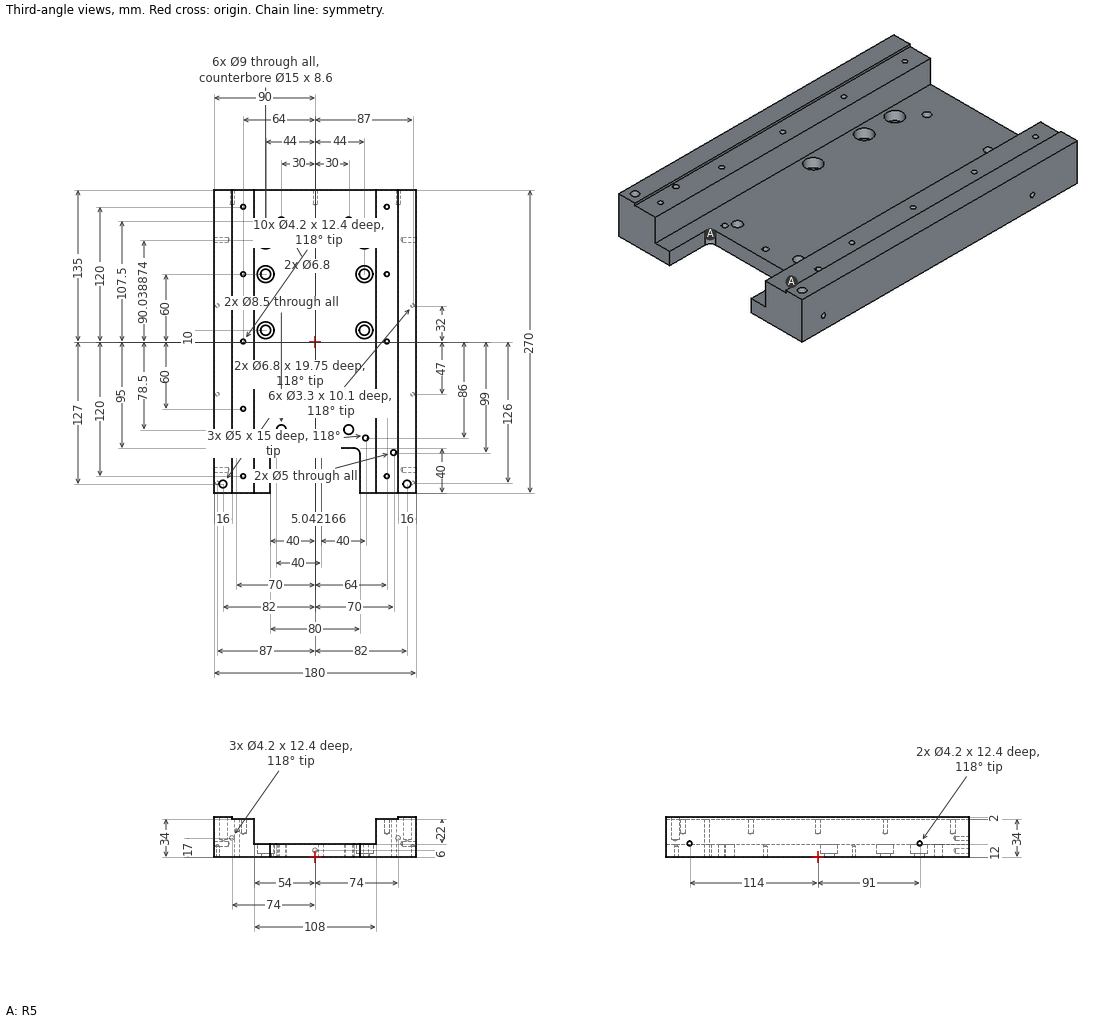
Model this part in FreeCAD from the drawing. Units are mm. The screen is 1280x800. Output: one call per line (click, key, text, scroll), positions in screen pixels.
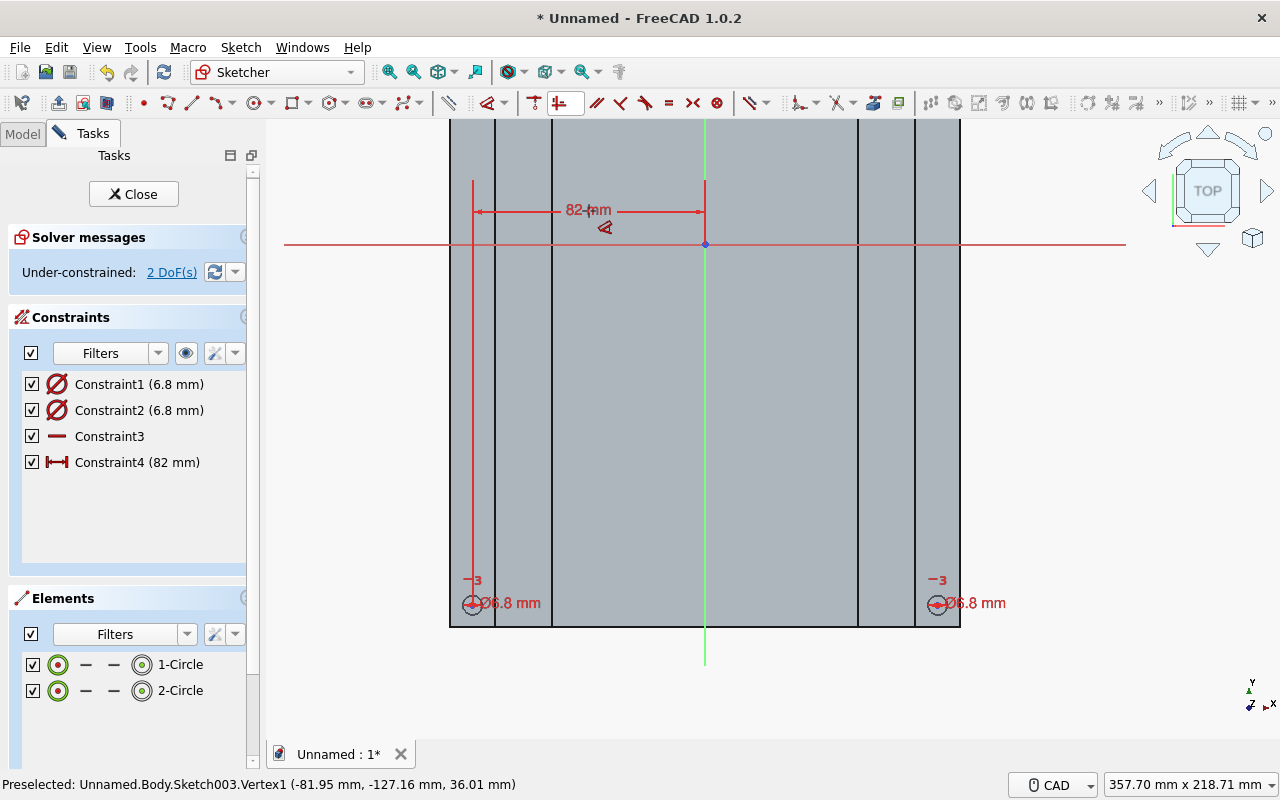
click(938, 605)
click(821, 211)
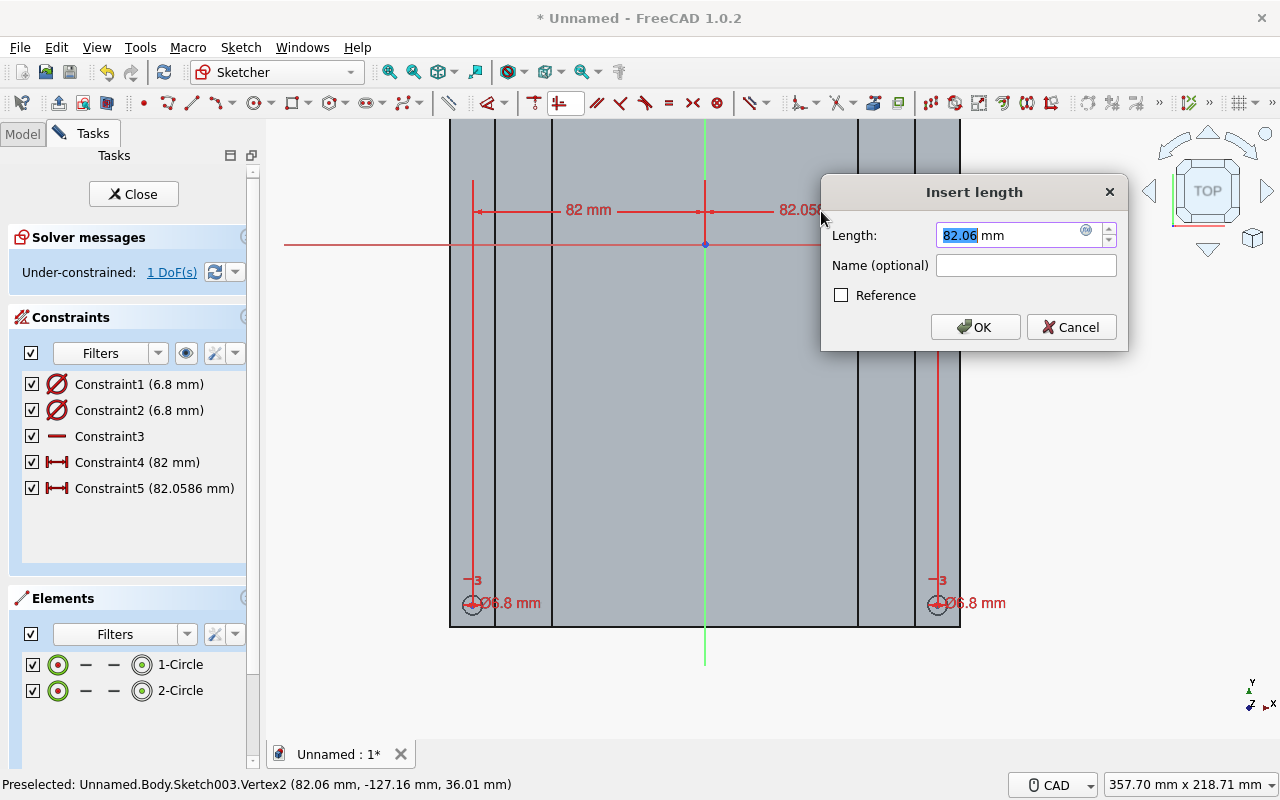
text(82)
key(Return)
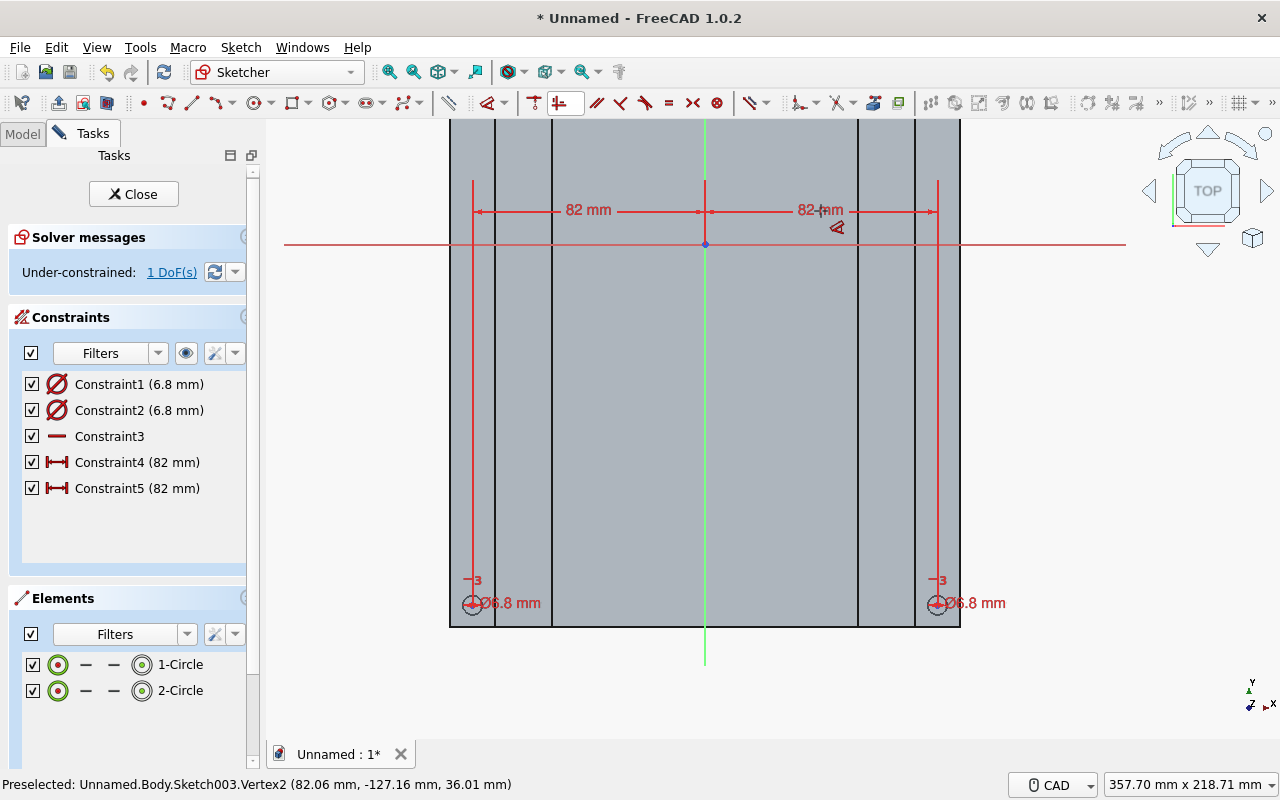
click(473, 605)
click(439, 425)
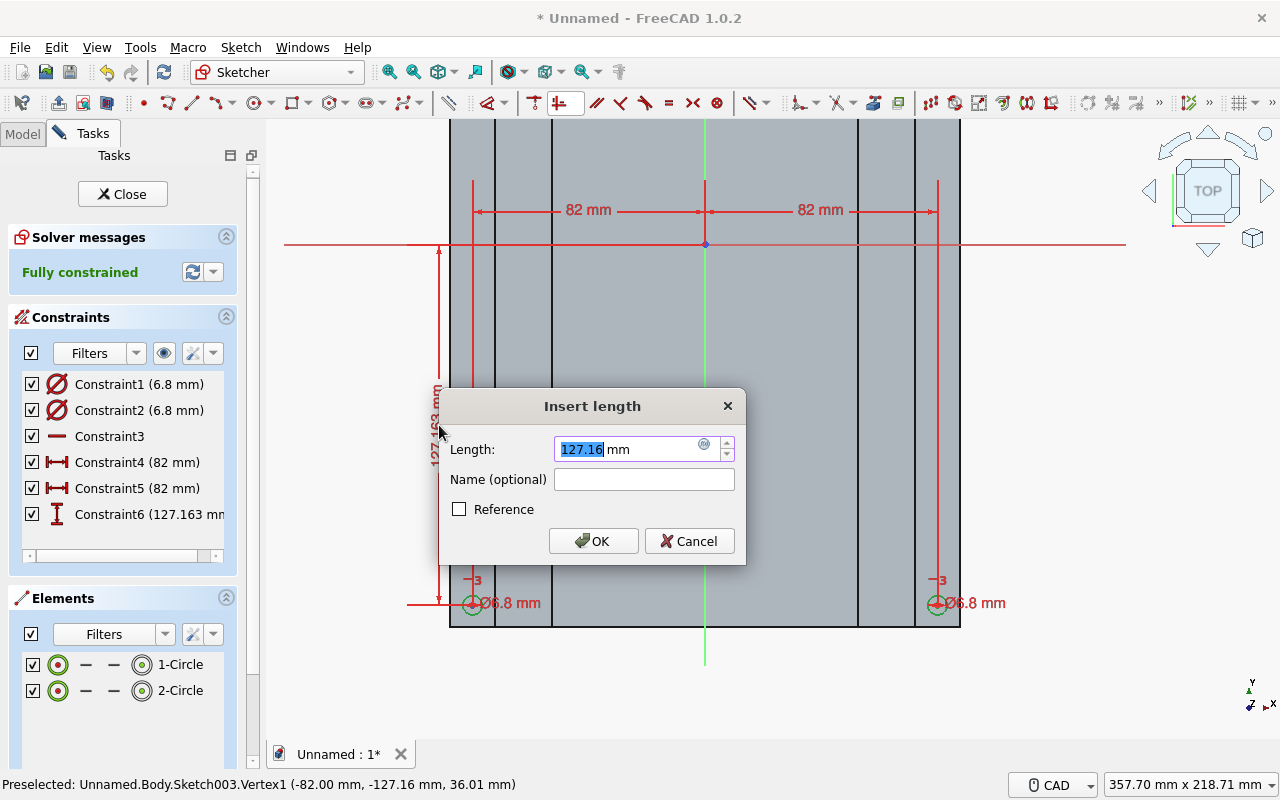
text(127)
key(Return)
key(Escape)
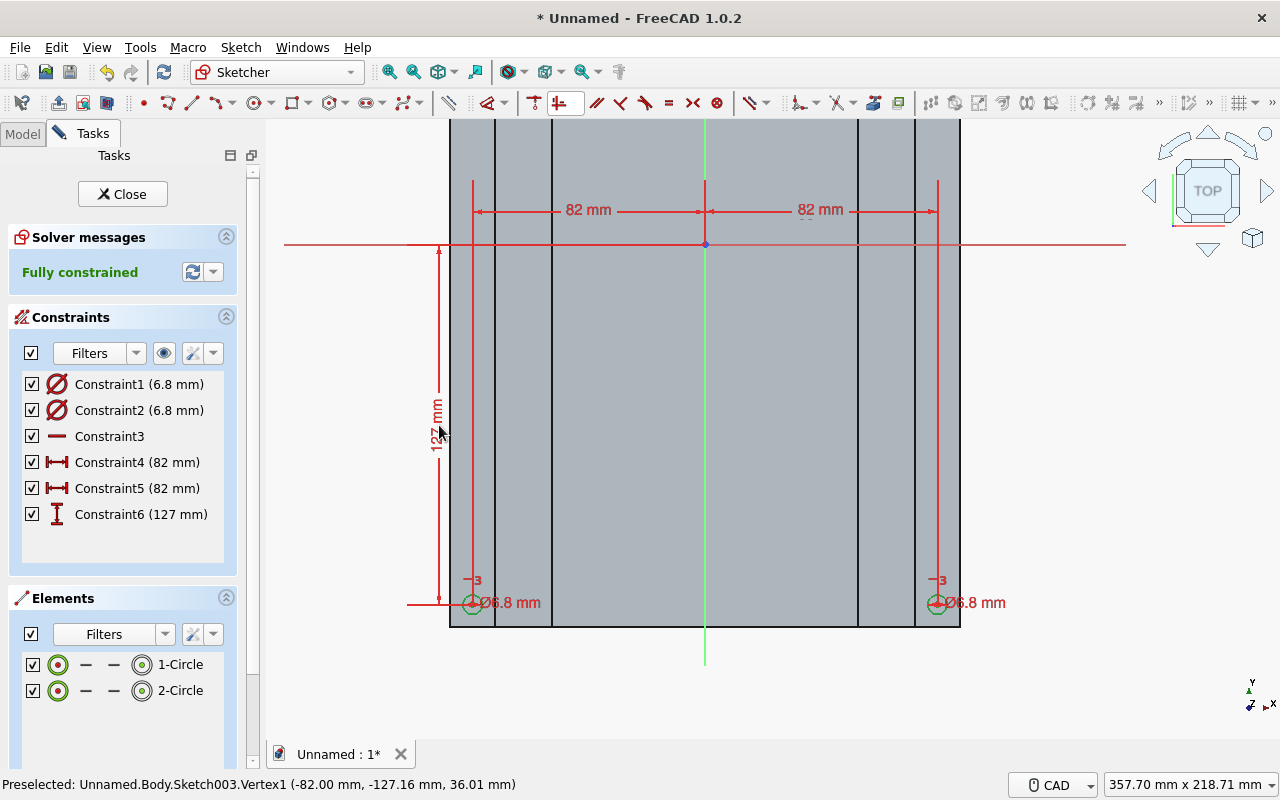
click(123, 194)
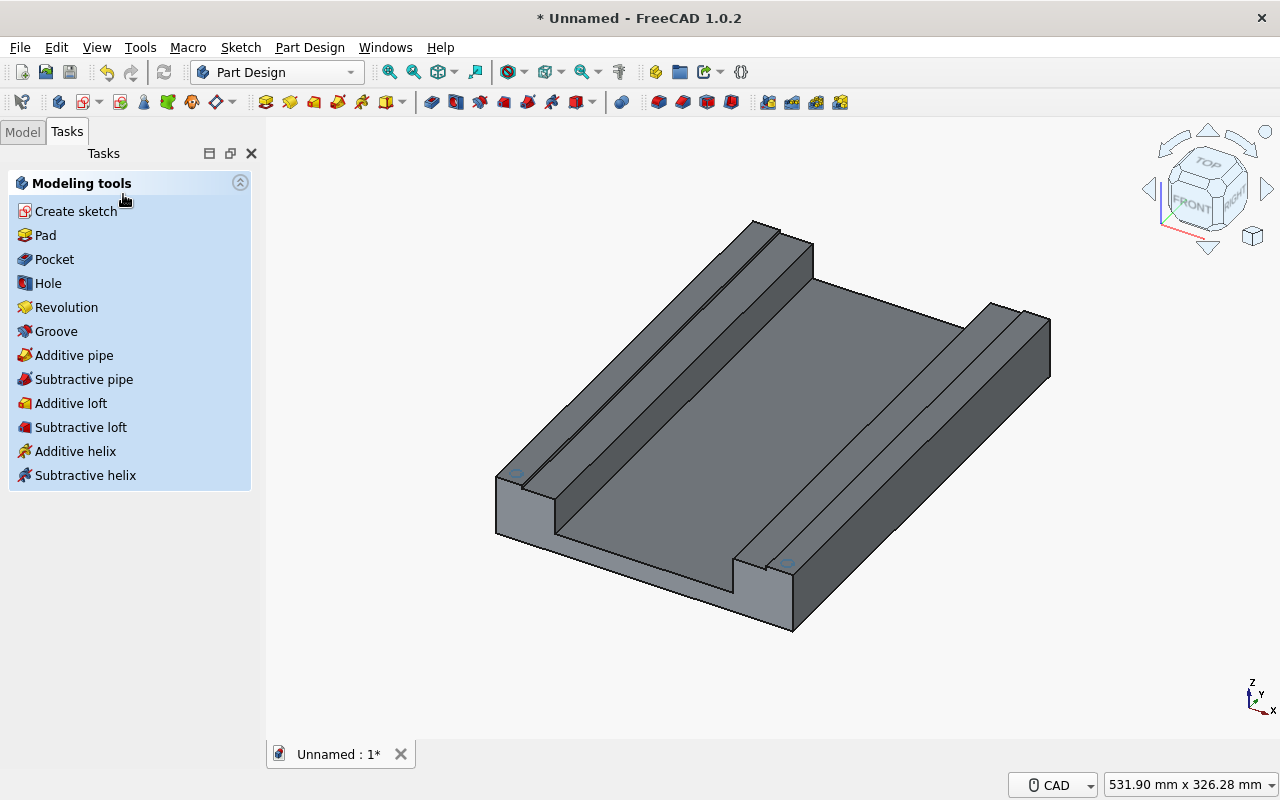
click(456, 102)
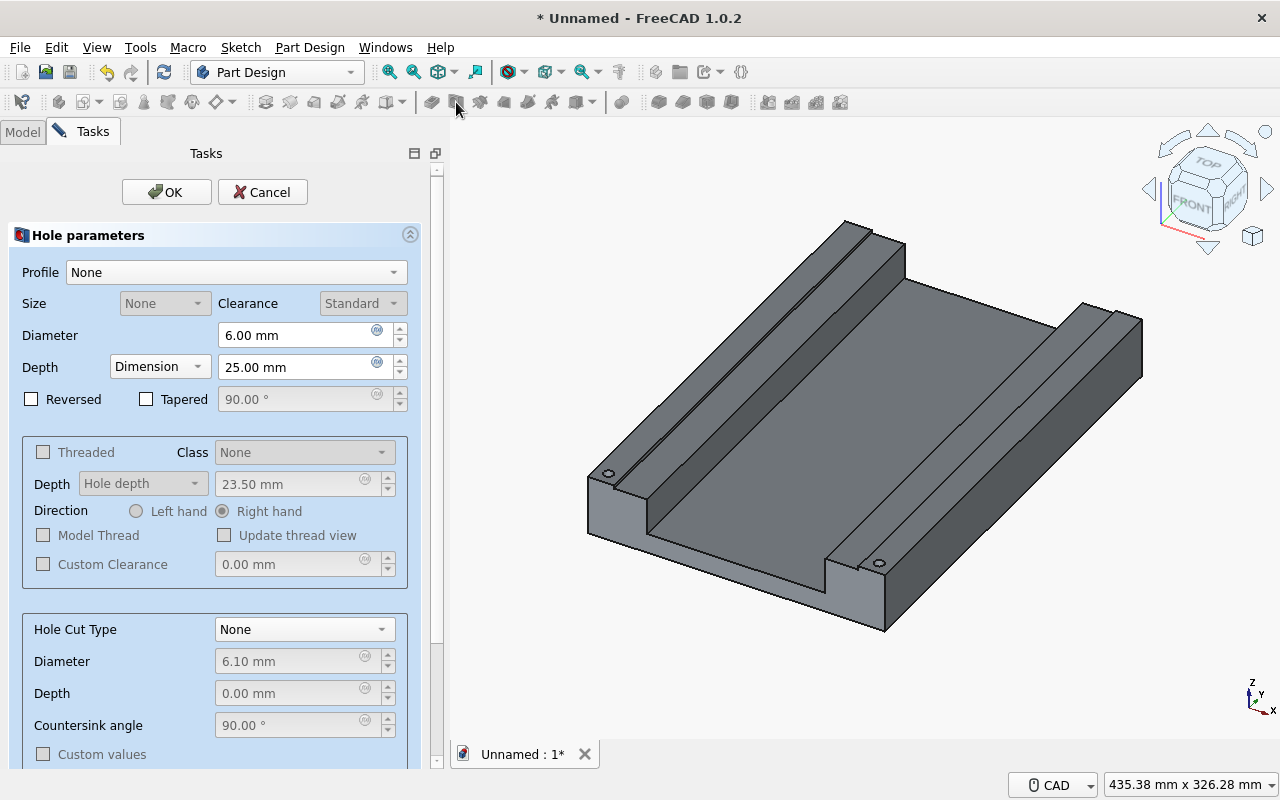
triple_click(305, 335)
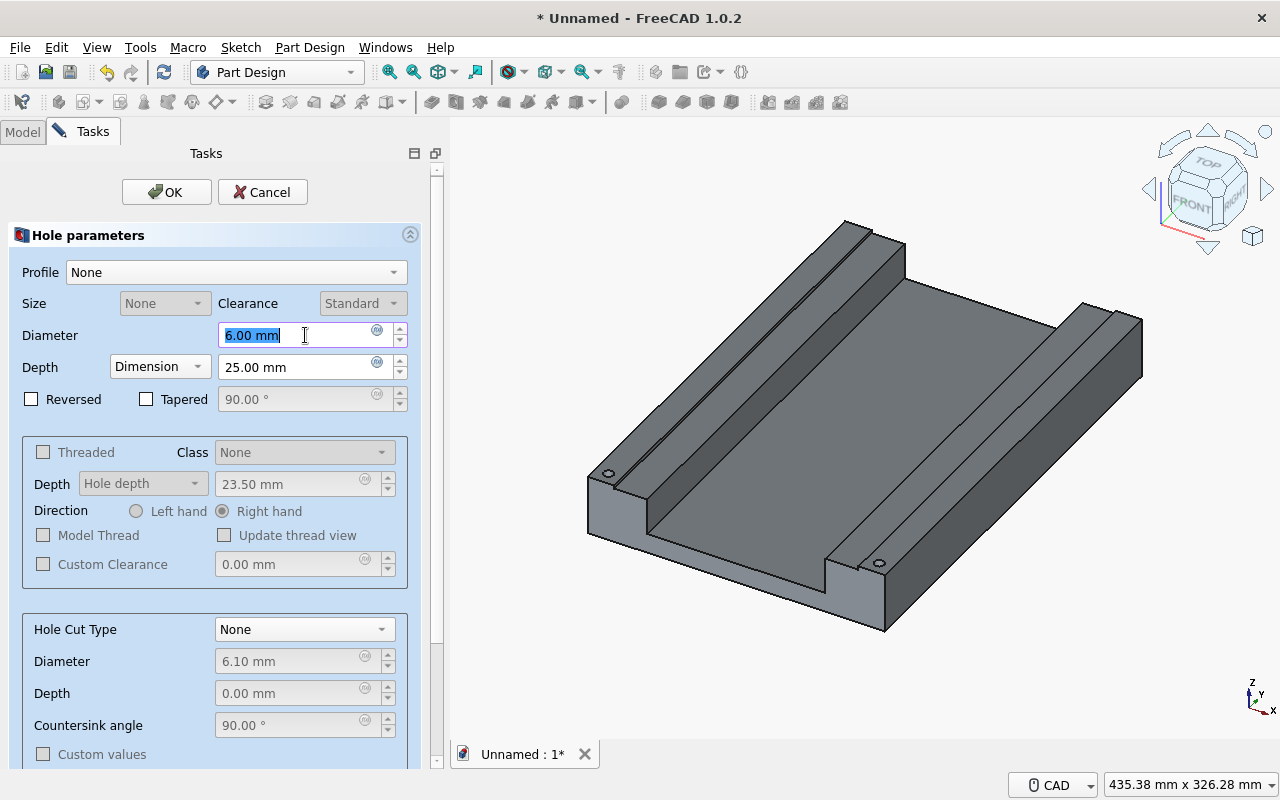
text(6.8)
key(Tab)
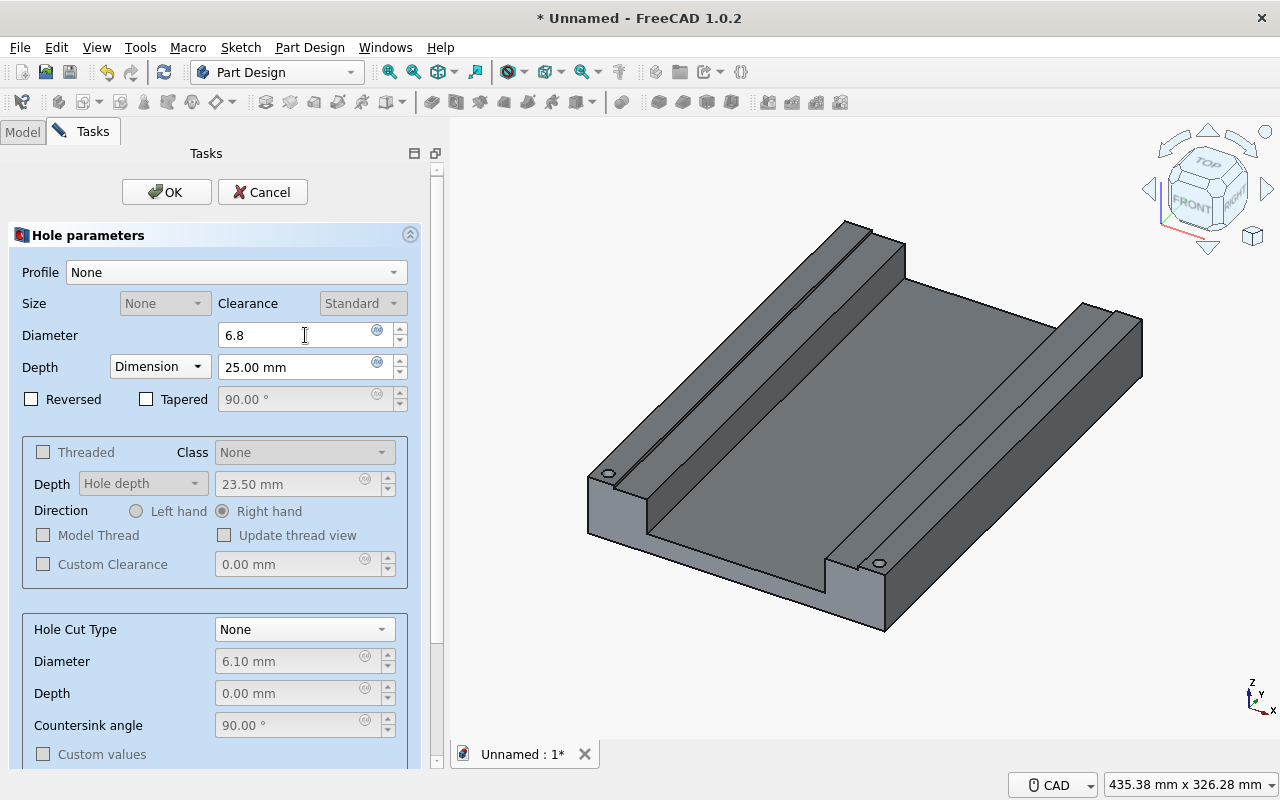
triple_click(305, 367)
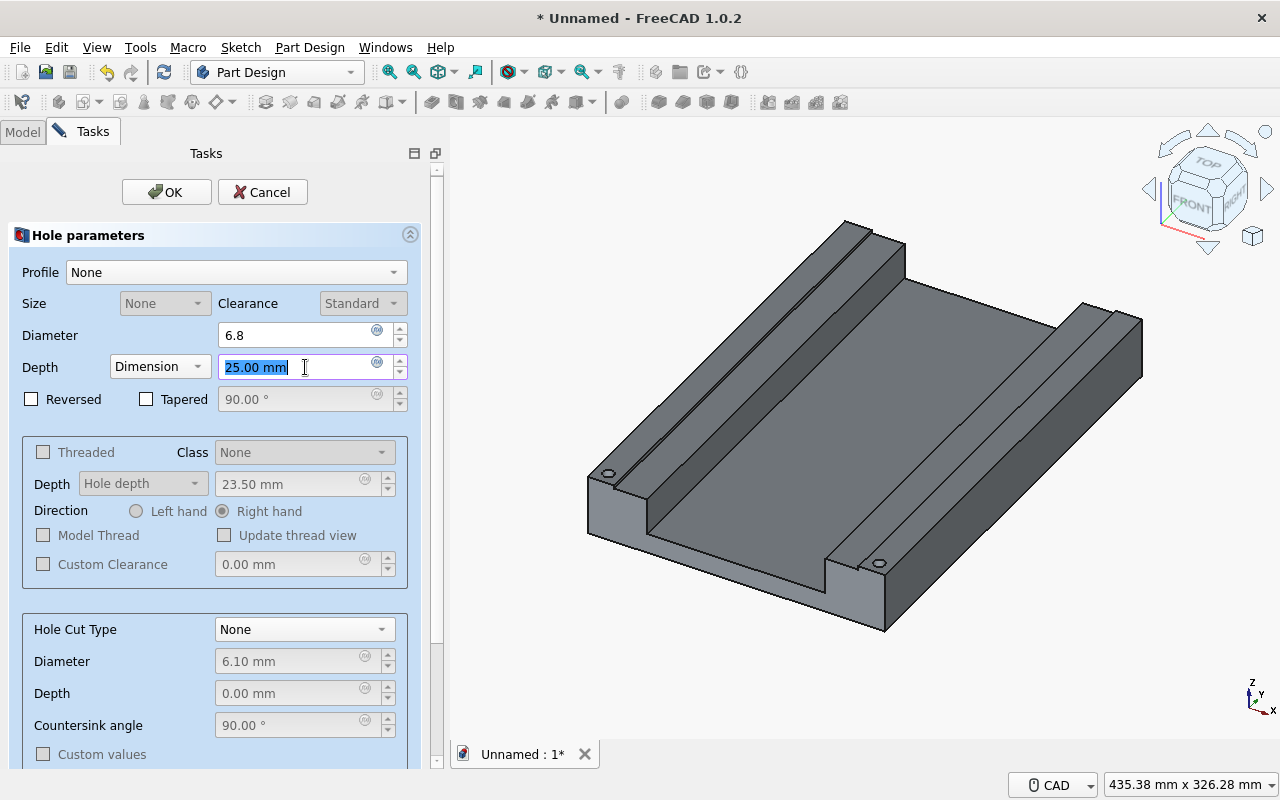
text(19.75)
key(Tab)